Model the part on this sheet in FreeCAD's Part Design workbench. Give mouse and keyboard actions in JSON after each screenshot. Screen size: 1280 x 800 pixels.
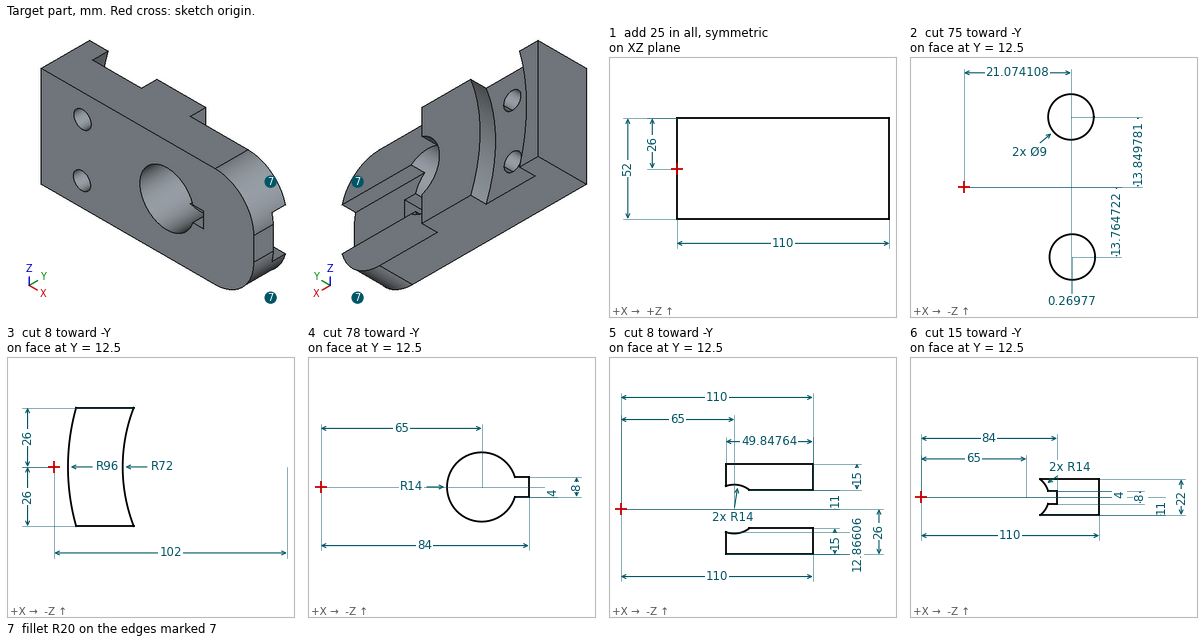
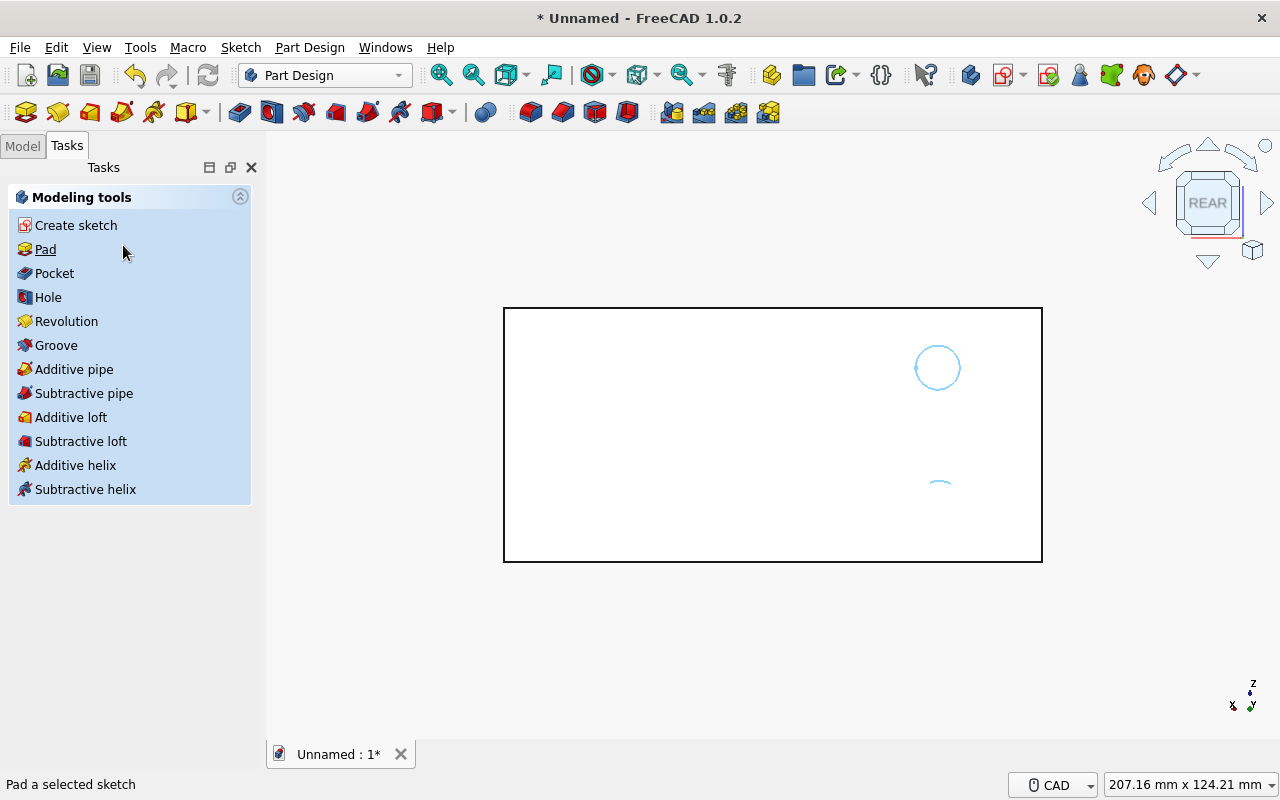
{"action": "left_click", "coordinate": [240, 112]}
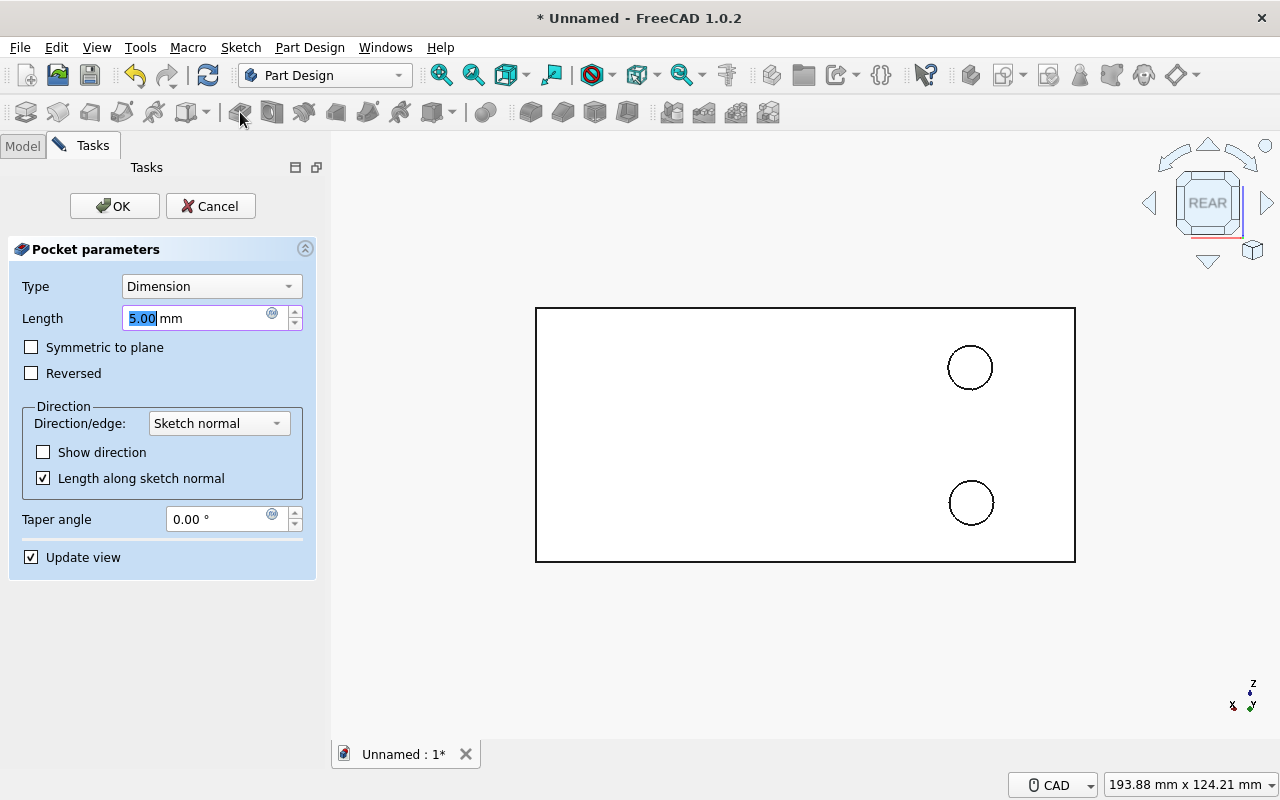
{"action": "type", "text": "75"}
{"action": "key", "text": "Tab"}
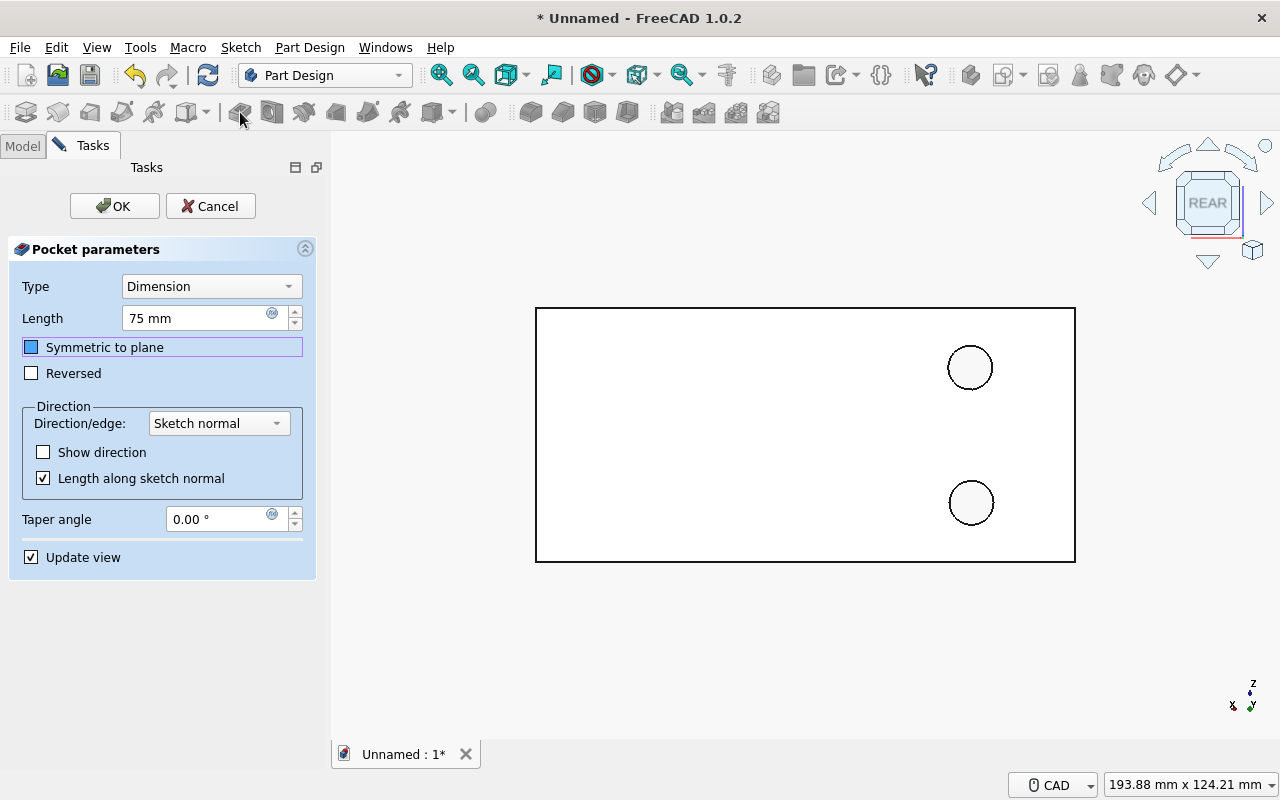
{"action": "left_click", "coordinate": [115, 206]}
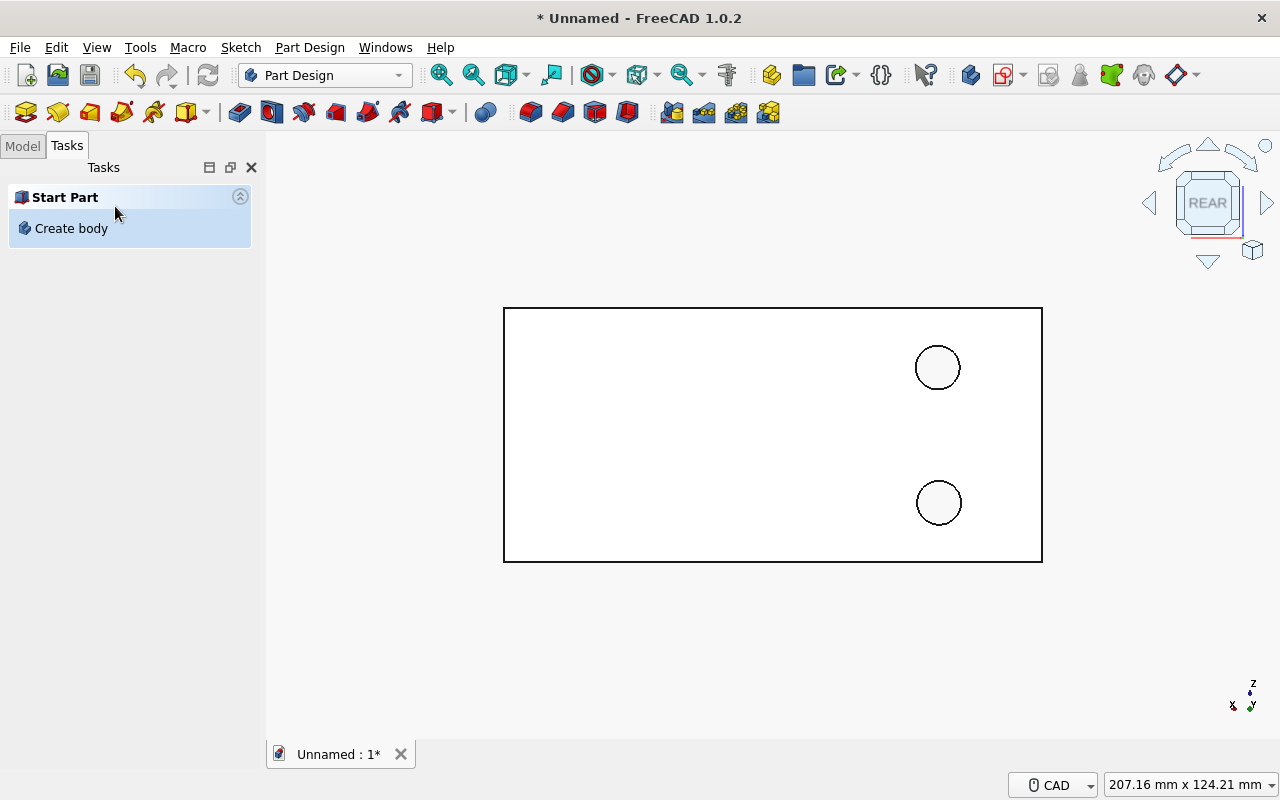
{"action": "left_click", "coordinate": [696, 434]}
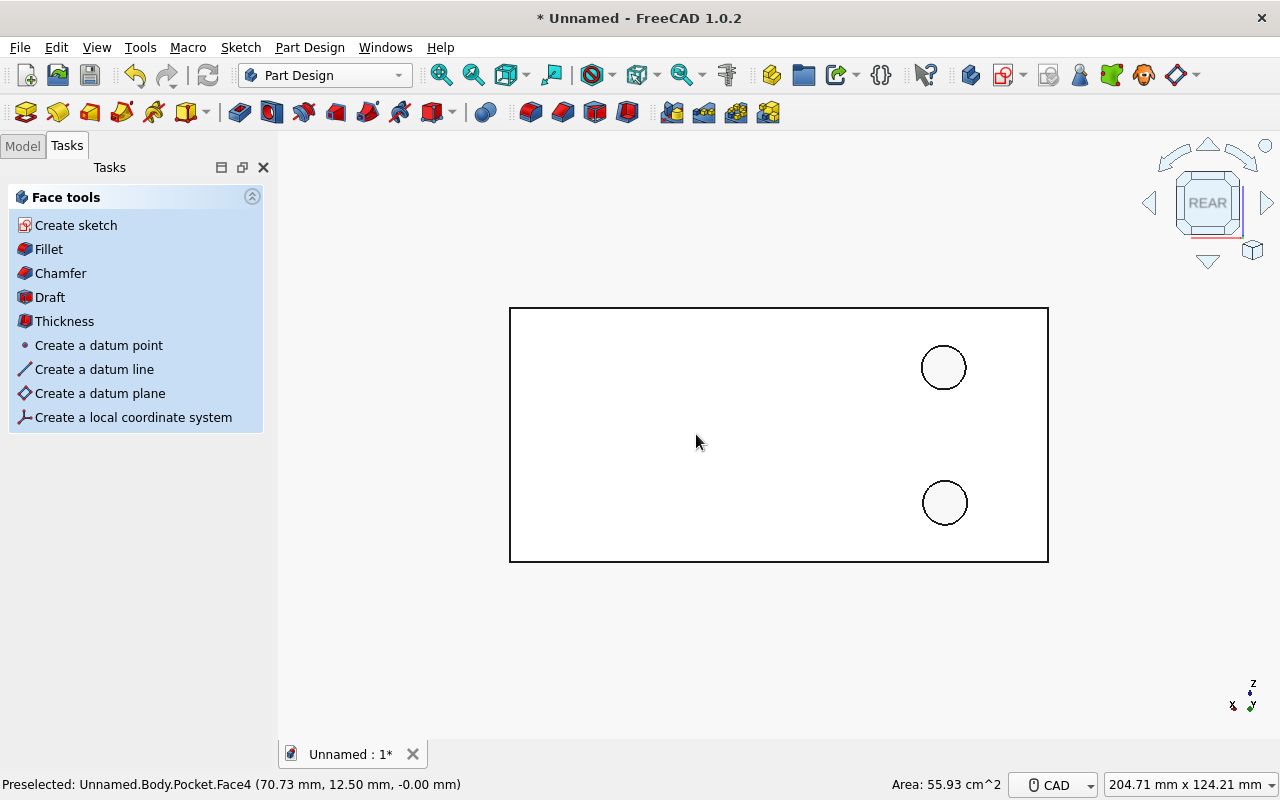
{"action": "left_click", "coordinate": [1004, 76]}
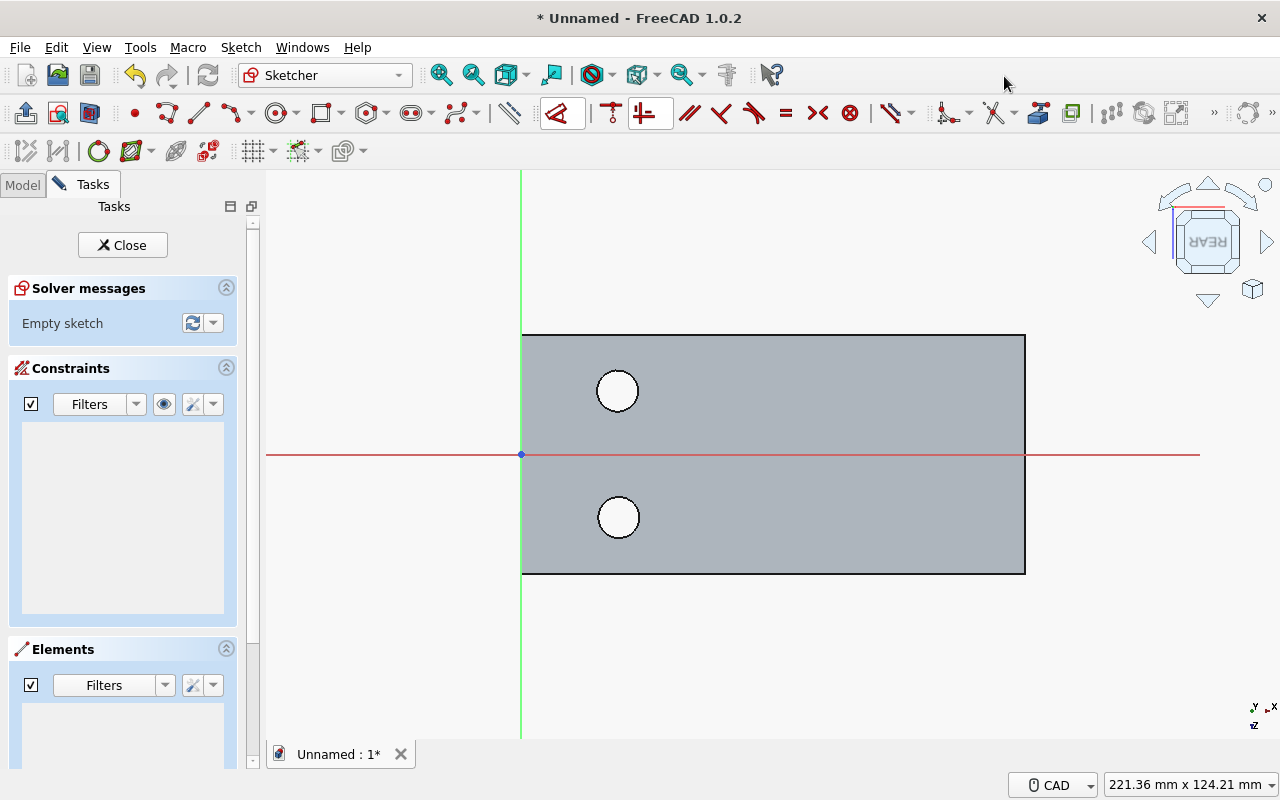
{"action": "scroll", "coordinate": [390, 454], "scroll_direction": "up", "scroll_amount": 2}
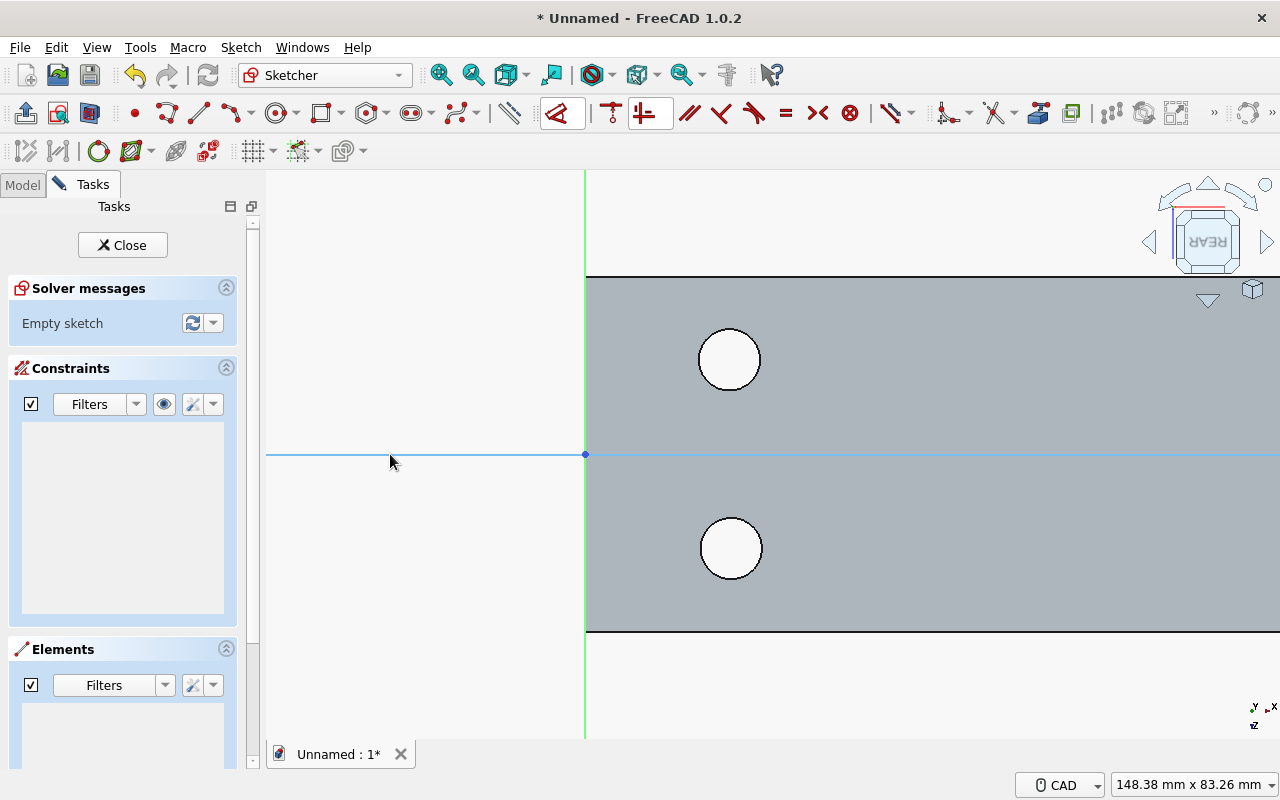
{"action": "left_click", "coordinate": [200, 114]}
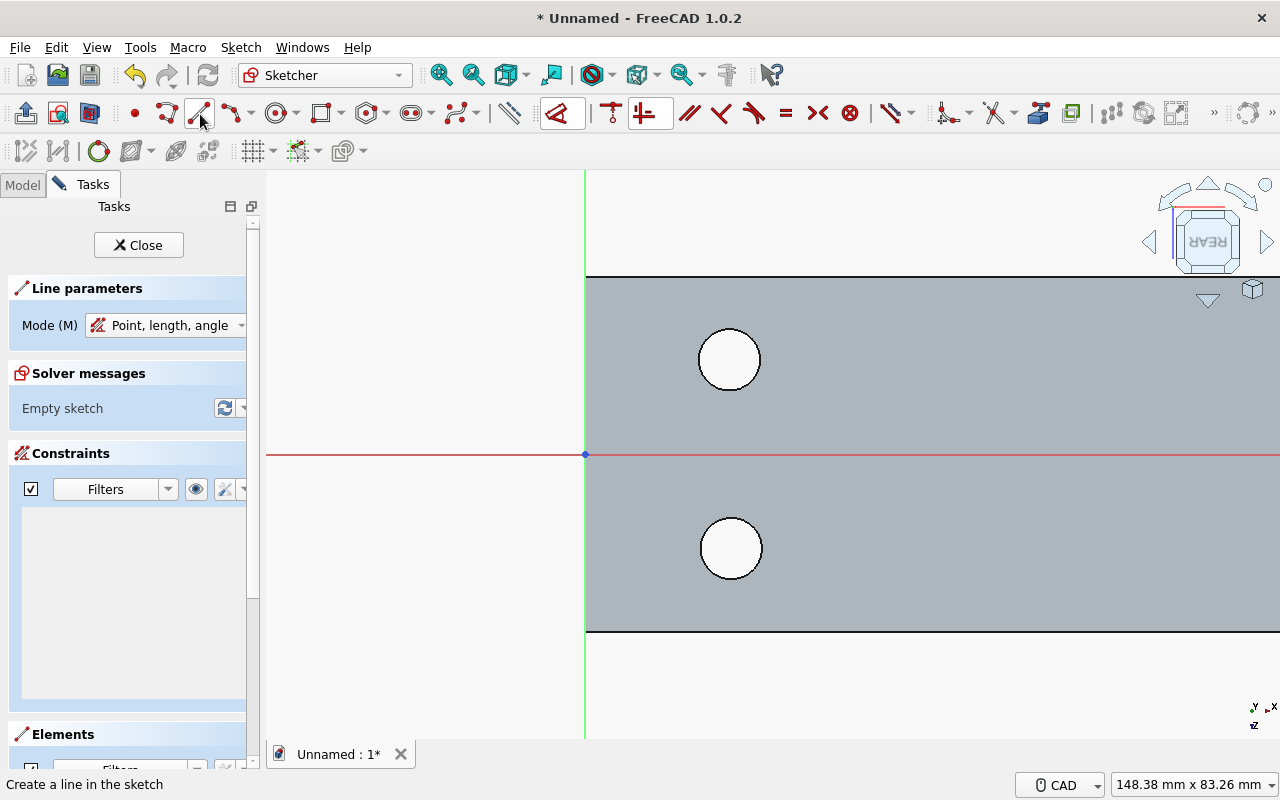
{"action": "left_click", "coordinate": [824, 277]}
{"action": "left_click", "coordinate": [651, 277]}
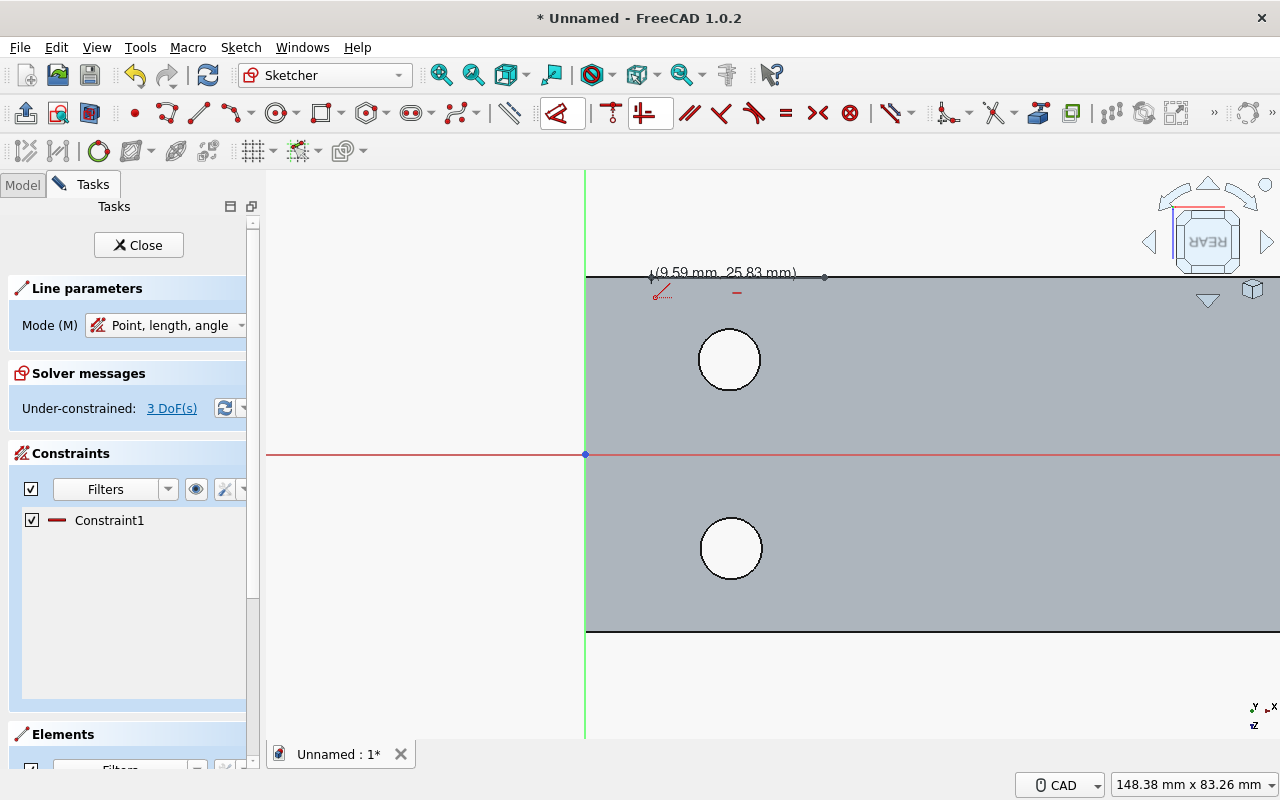
{"action": "left_click", "coordinate": [651, 632]}
{"action": "left_click", "coordinate": [824, 632]}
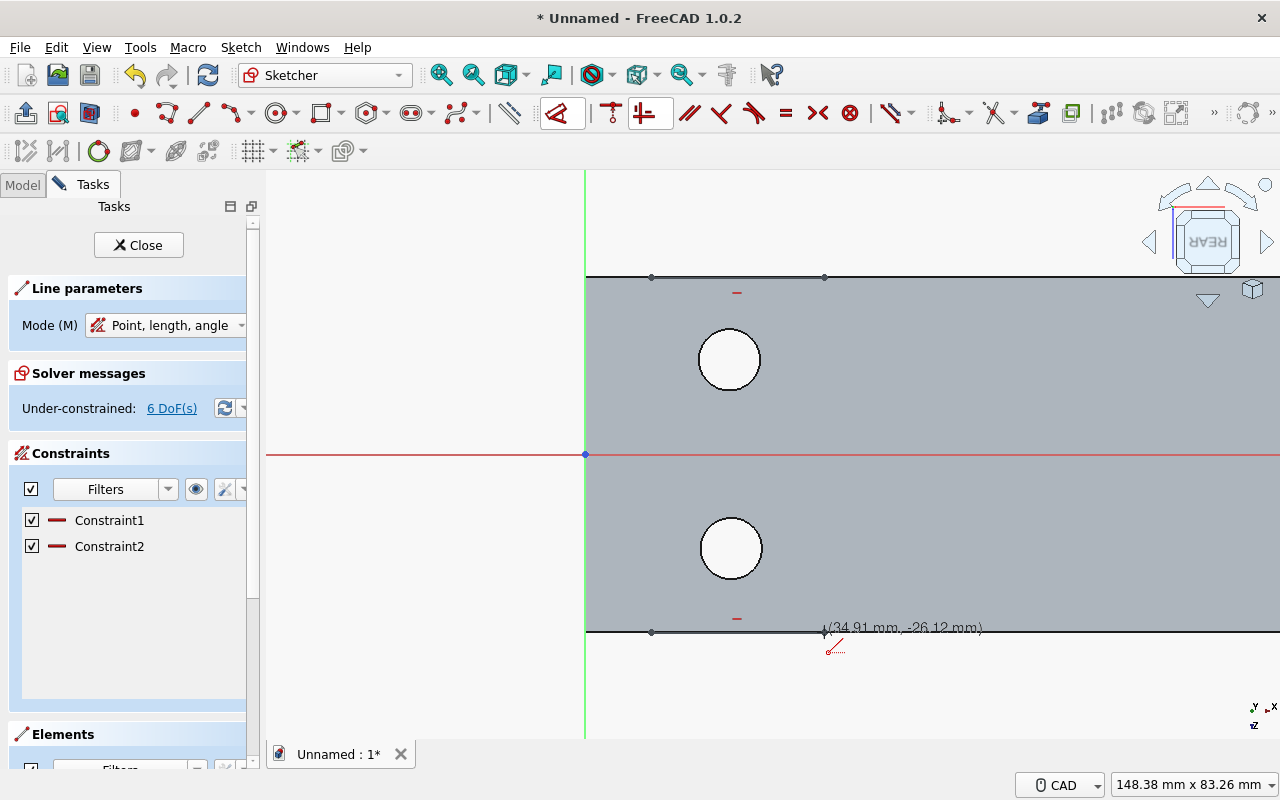
{"action": "left_click", "coordinate": [232, 114]}